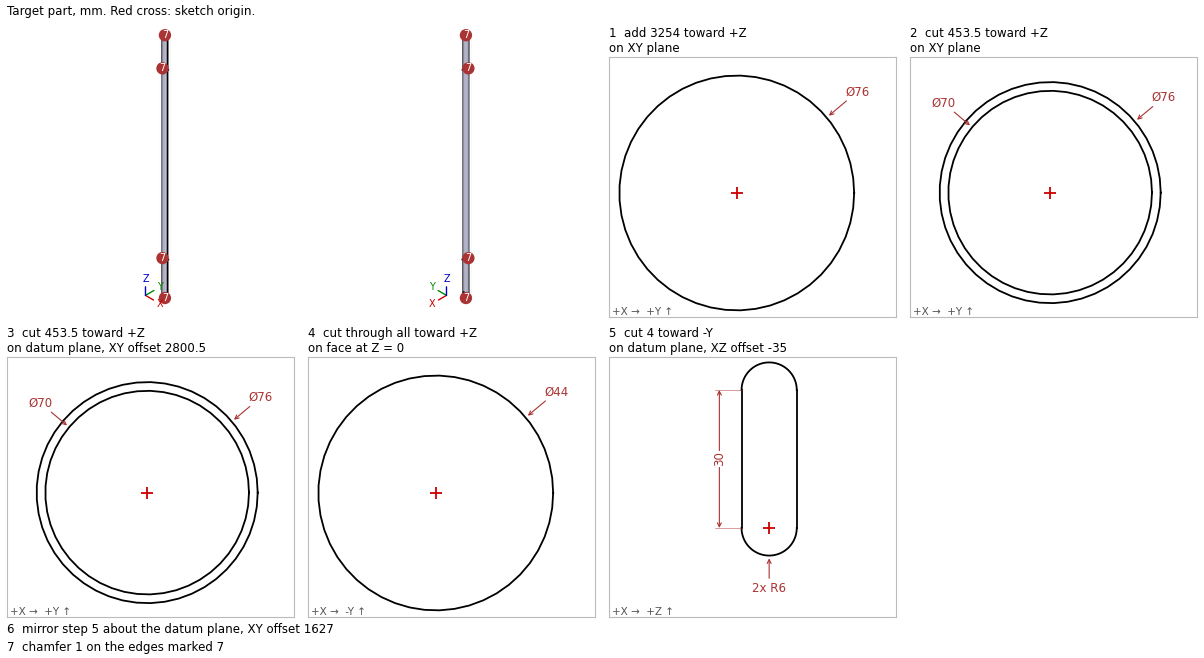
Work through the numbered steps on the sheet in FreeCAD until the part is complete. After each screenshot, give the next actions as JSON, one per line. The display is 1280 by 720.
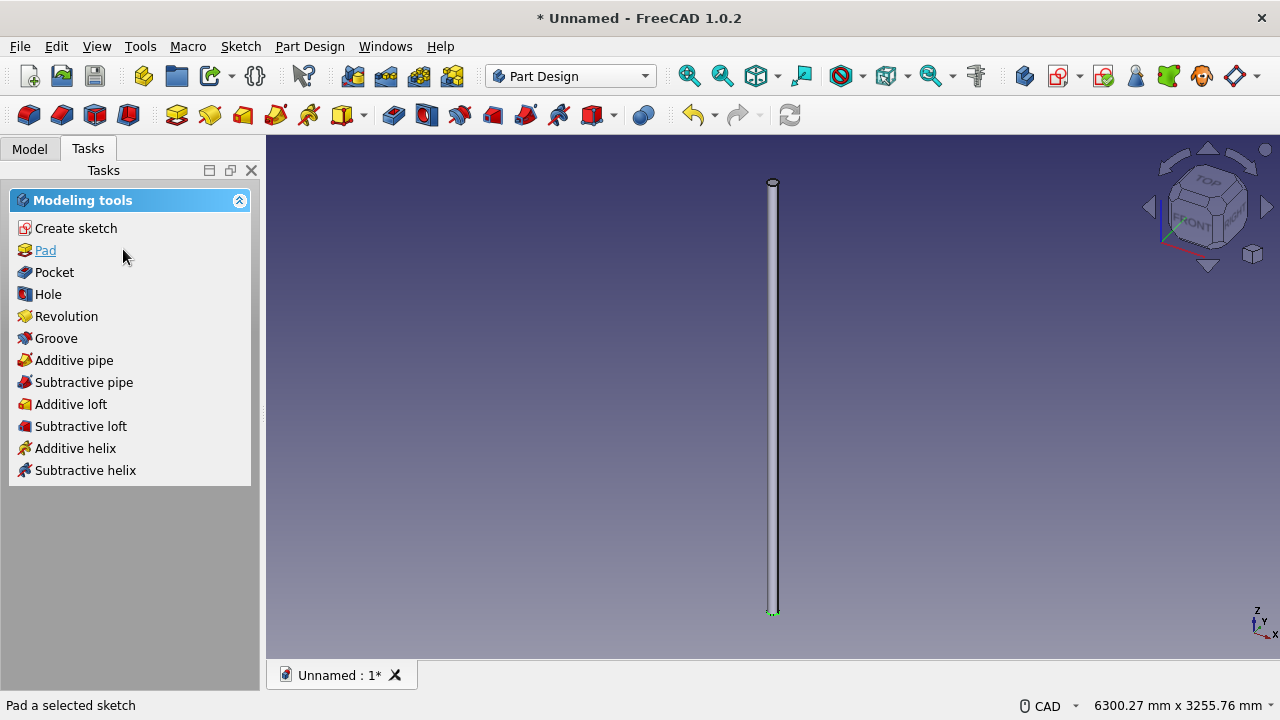
{"action": "left_click", "coordinate": [394, 116]}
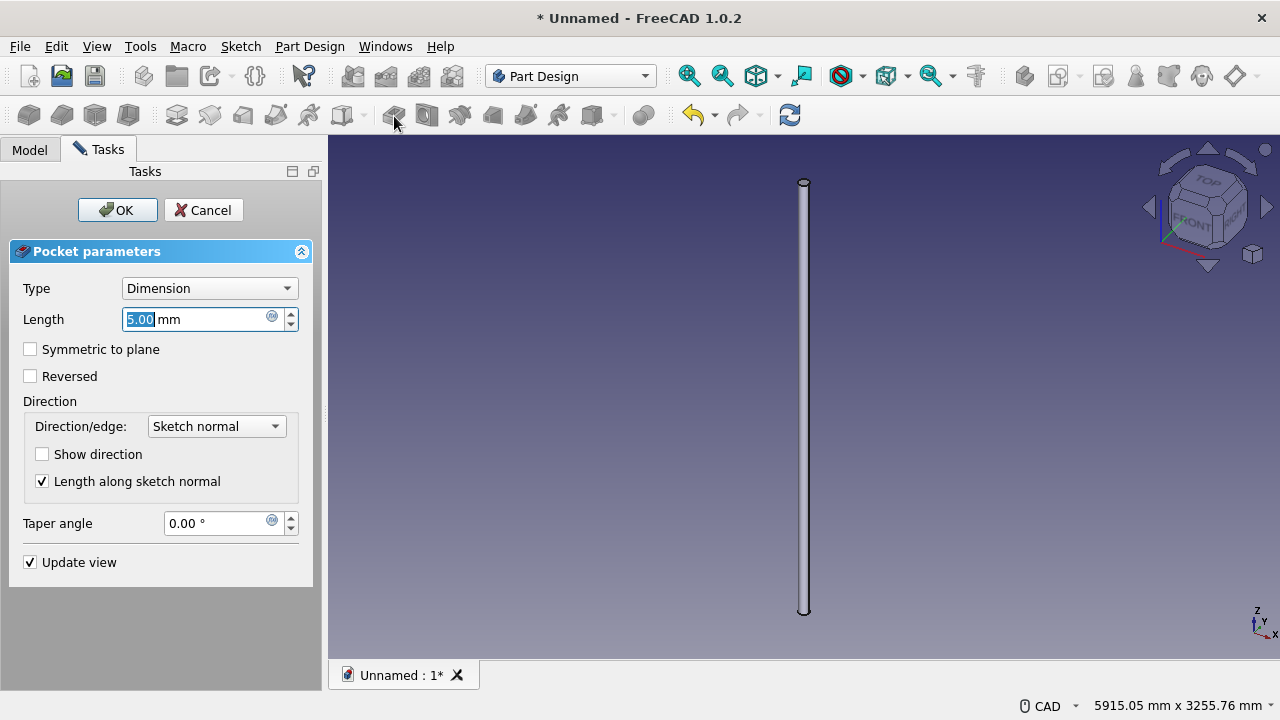
{"action": "type", "text": "453.5"}
{"action": "key", "text": "Tab"}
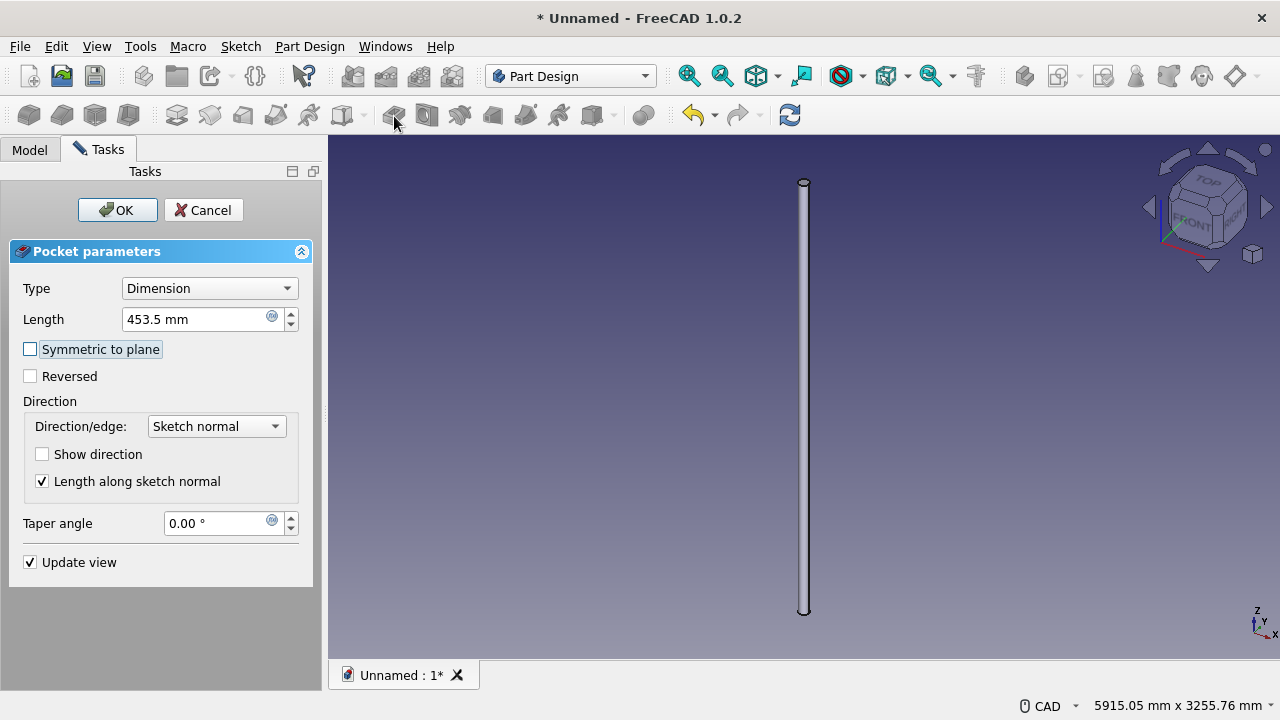
{"action": "left_click", "coordinate": [31, 376]}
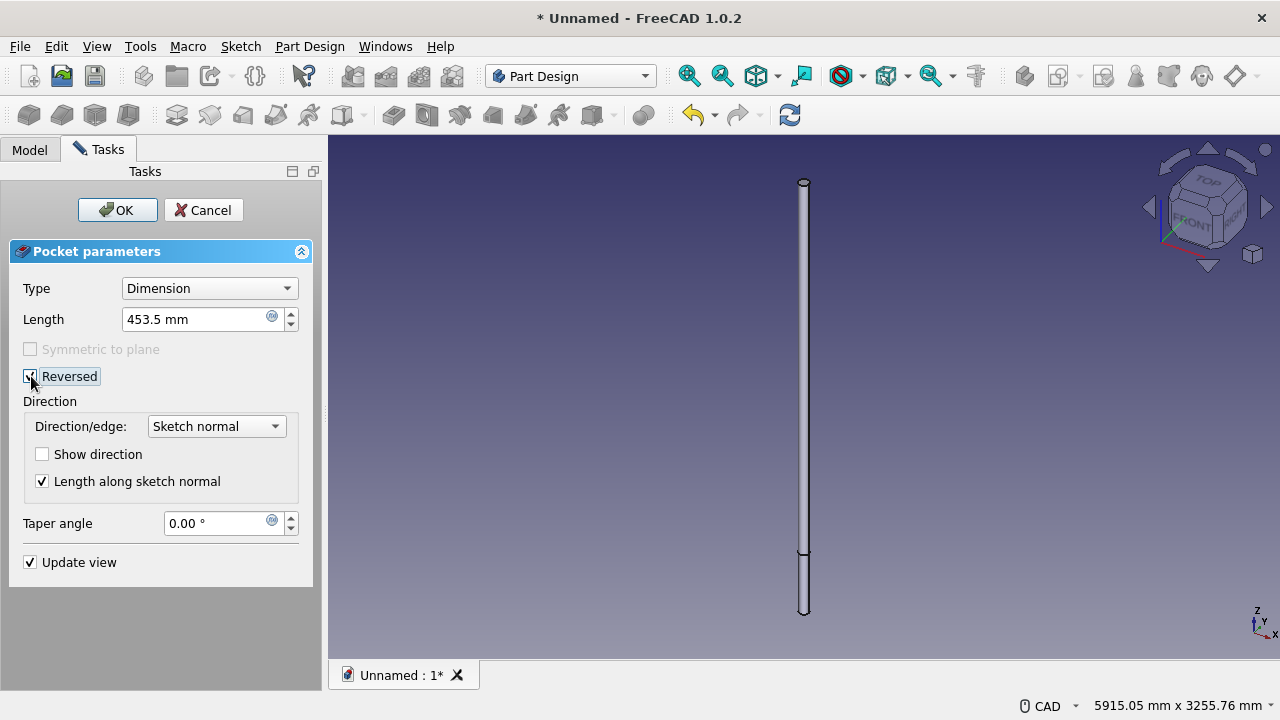
{"action": "left_click", "coordinate": [118, 210]}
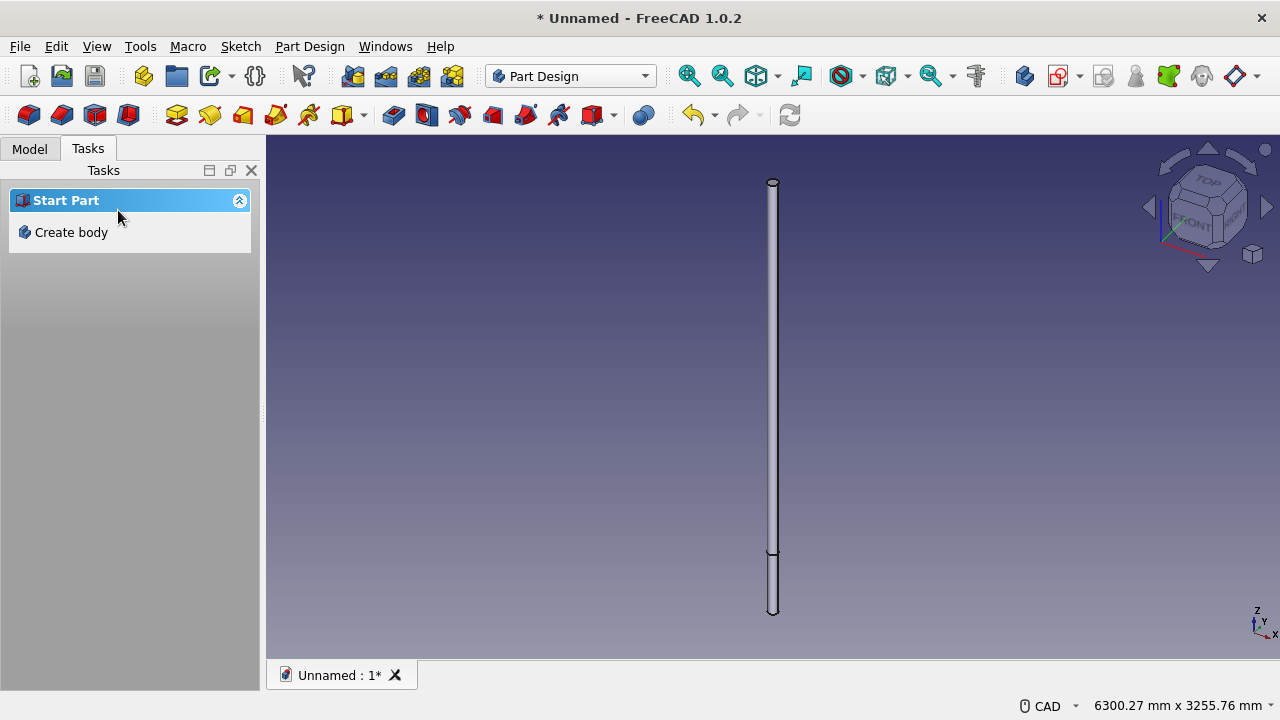
{"action": "left_click", "coordinate": [30, 148]}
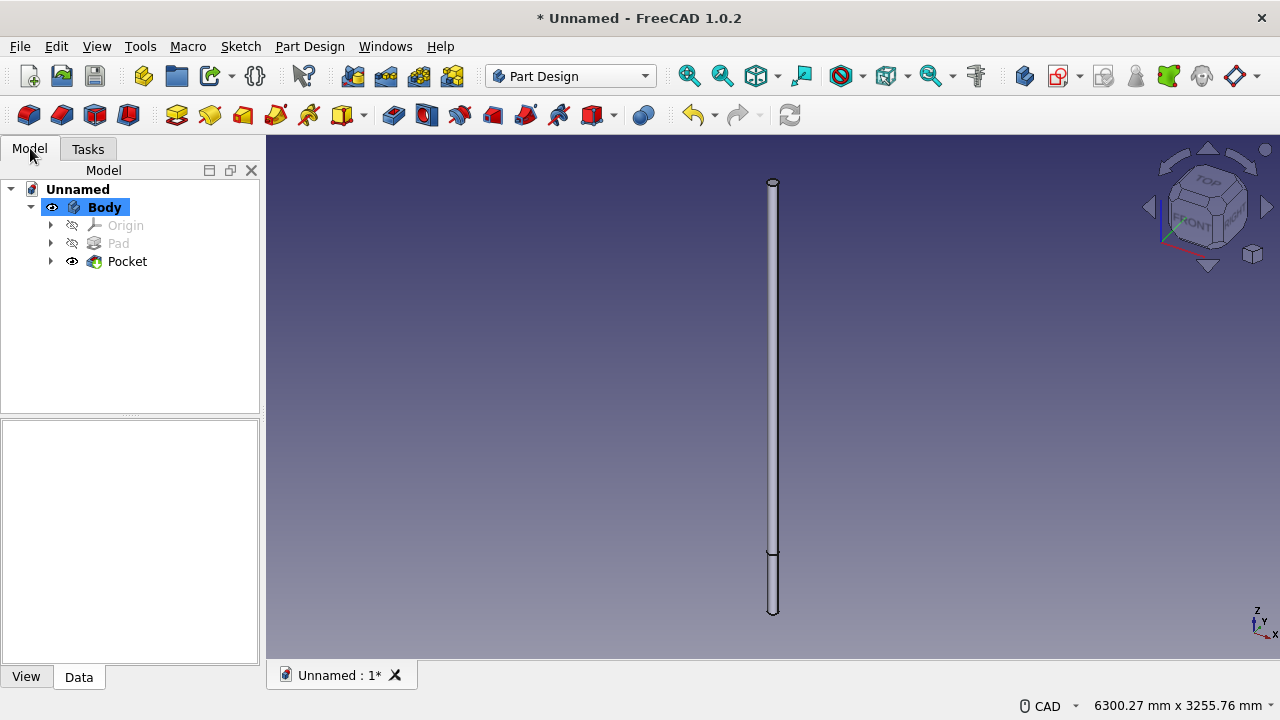
{"action": "left_click", "coordinate": [51, 225]}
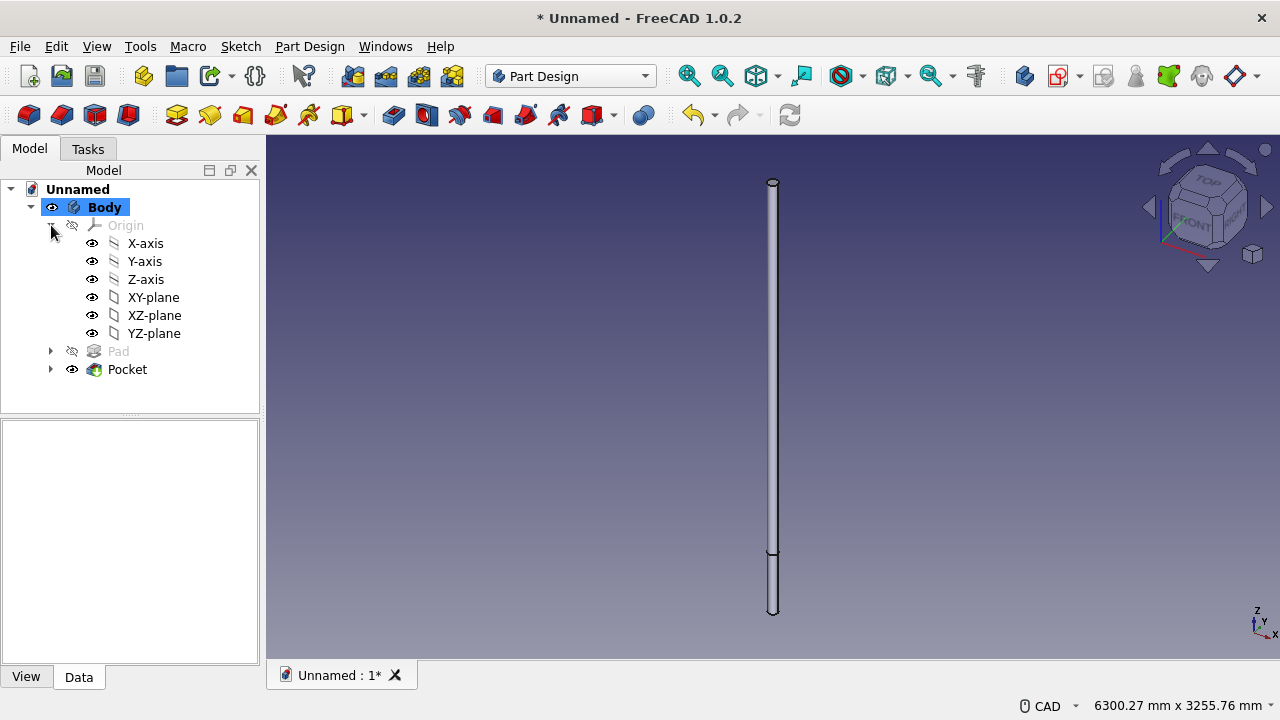
{"action": "left_click", "coordinate": [137, 297]}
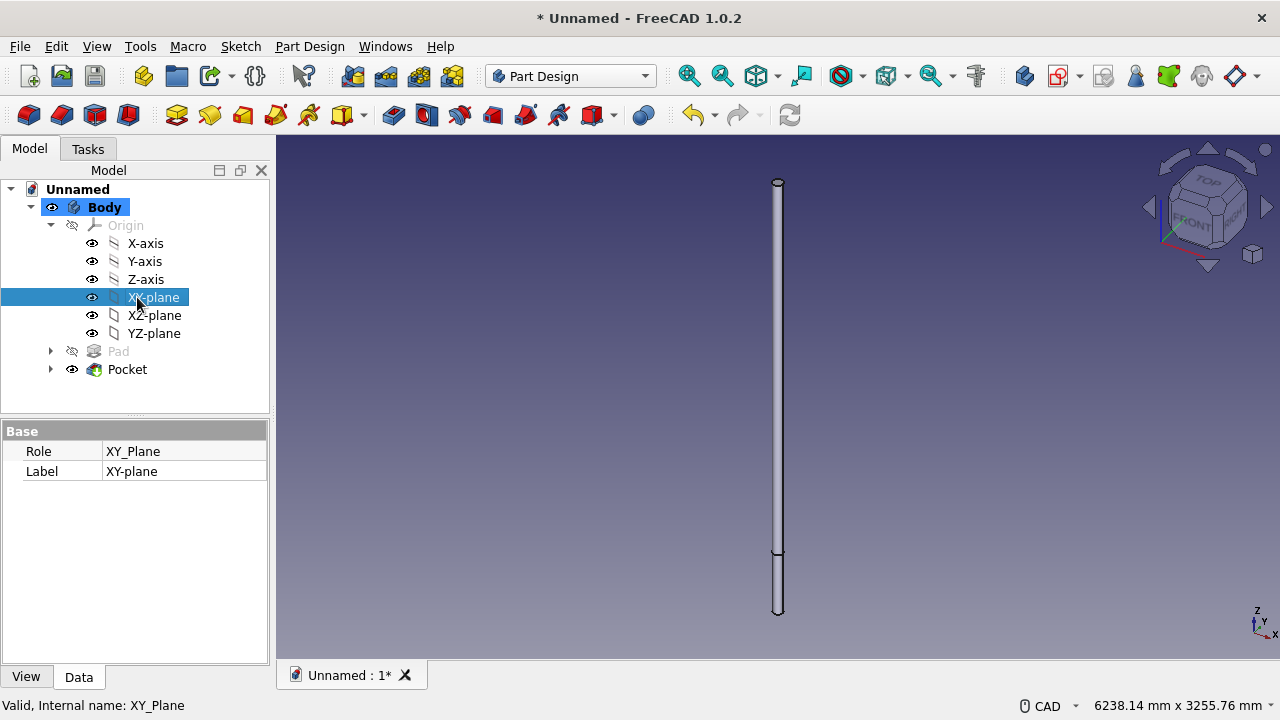
{"action": "left_click", "coordinate": [1234, 76]}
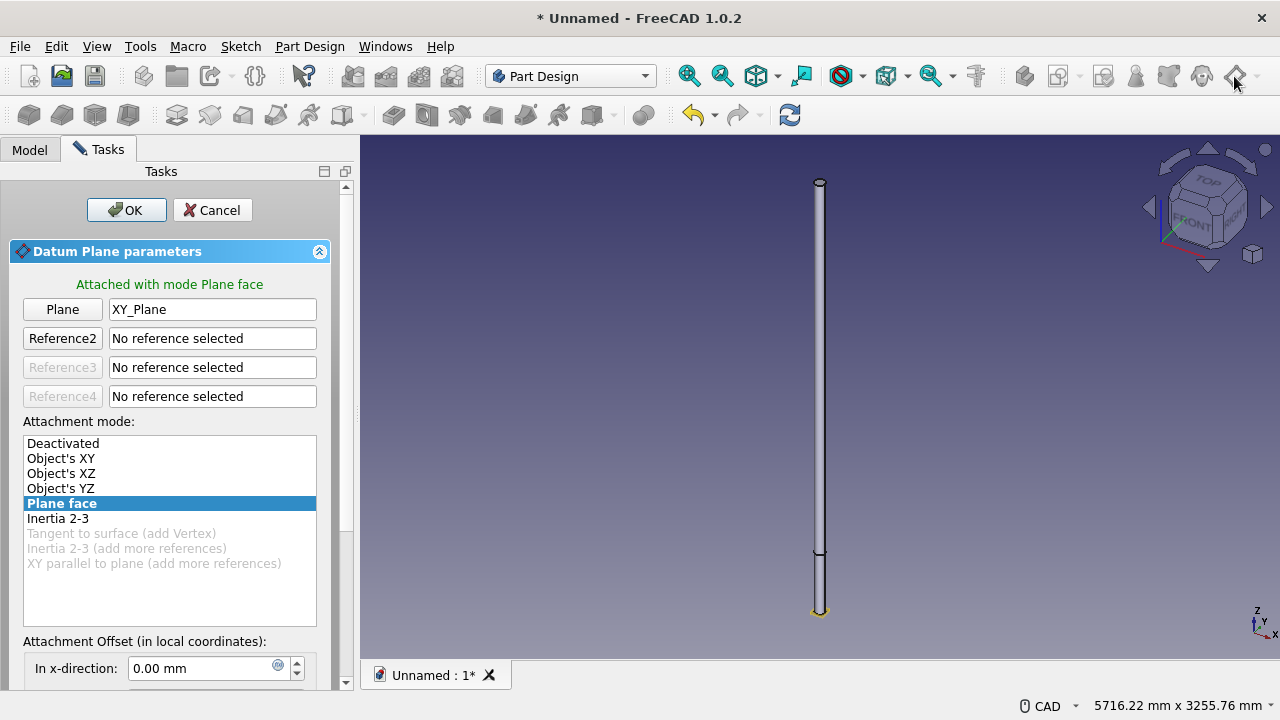
{"action": "scroll", "coordinate": [346, 436], "scroll_direction": "down", "scroll_amount": 2}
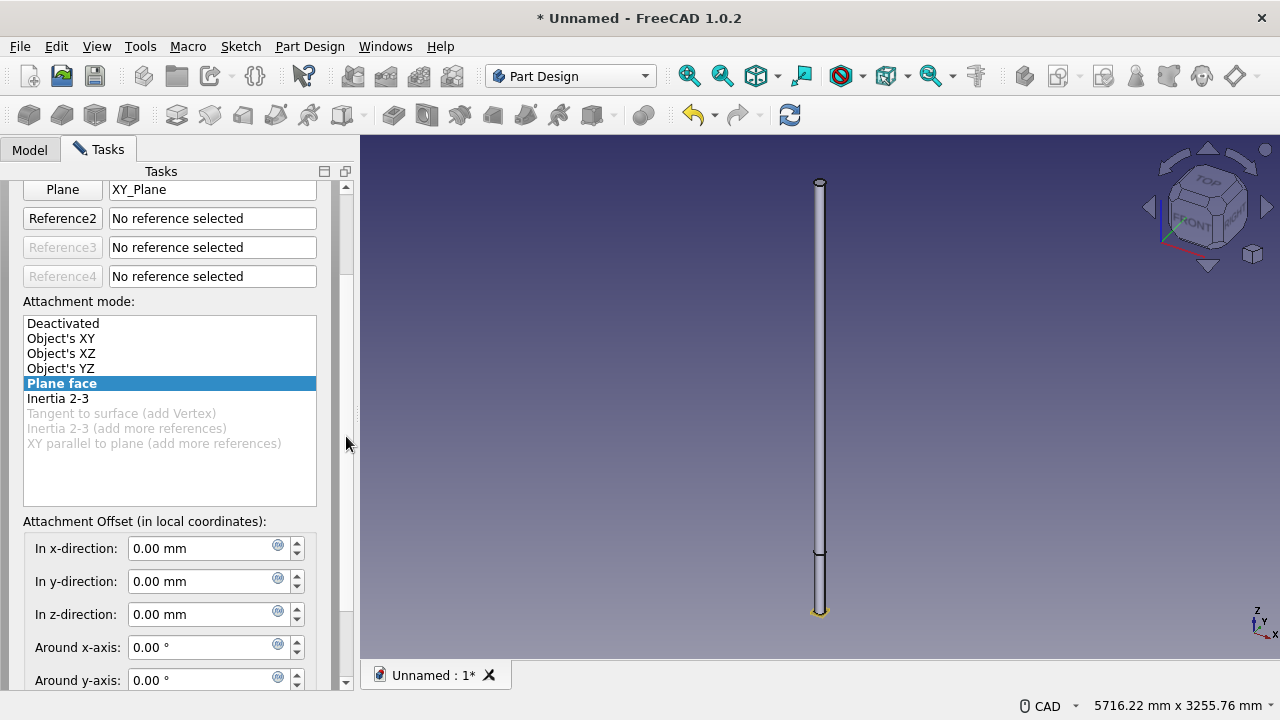
{"action": "triple_click", "coordinate": [210, 614]}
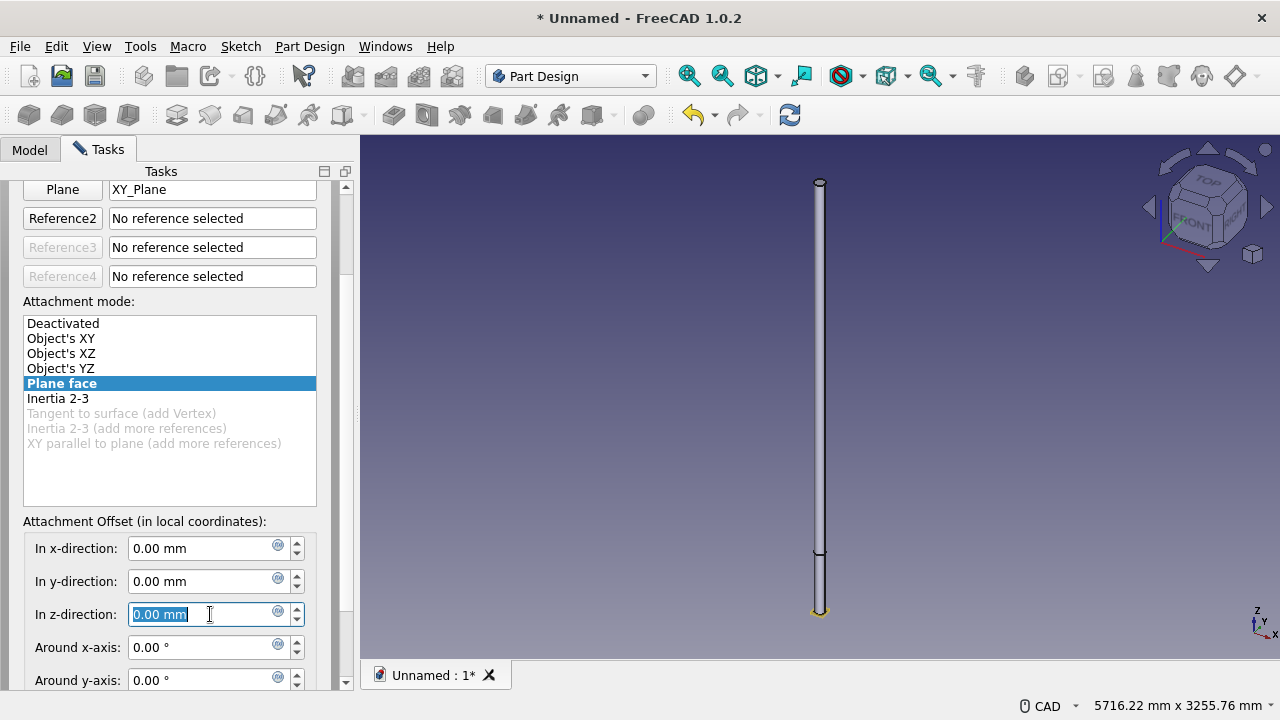
{"action": "type", "text": "2800.5"}
{"action": "key", "text": "Tab"}